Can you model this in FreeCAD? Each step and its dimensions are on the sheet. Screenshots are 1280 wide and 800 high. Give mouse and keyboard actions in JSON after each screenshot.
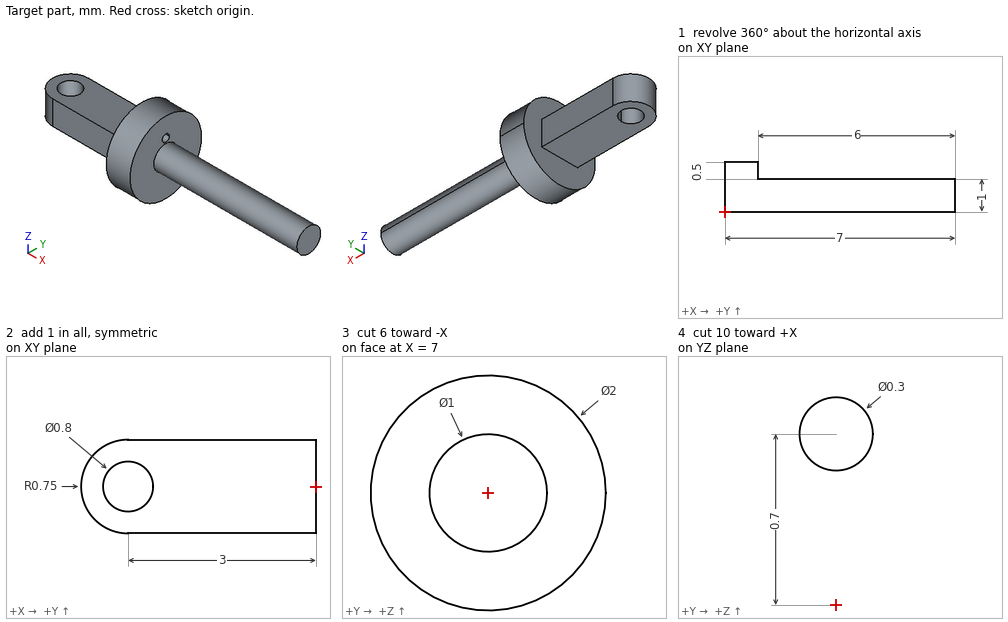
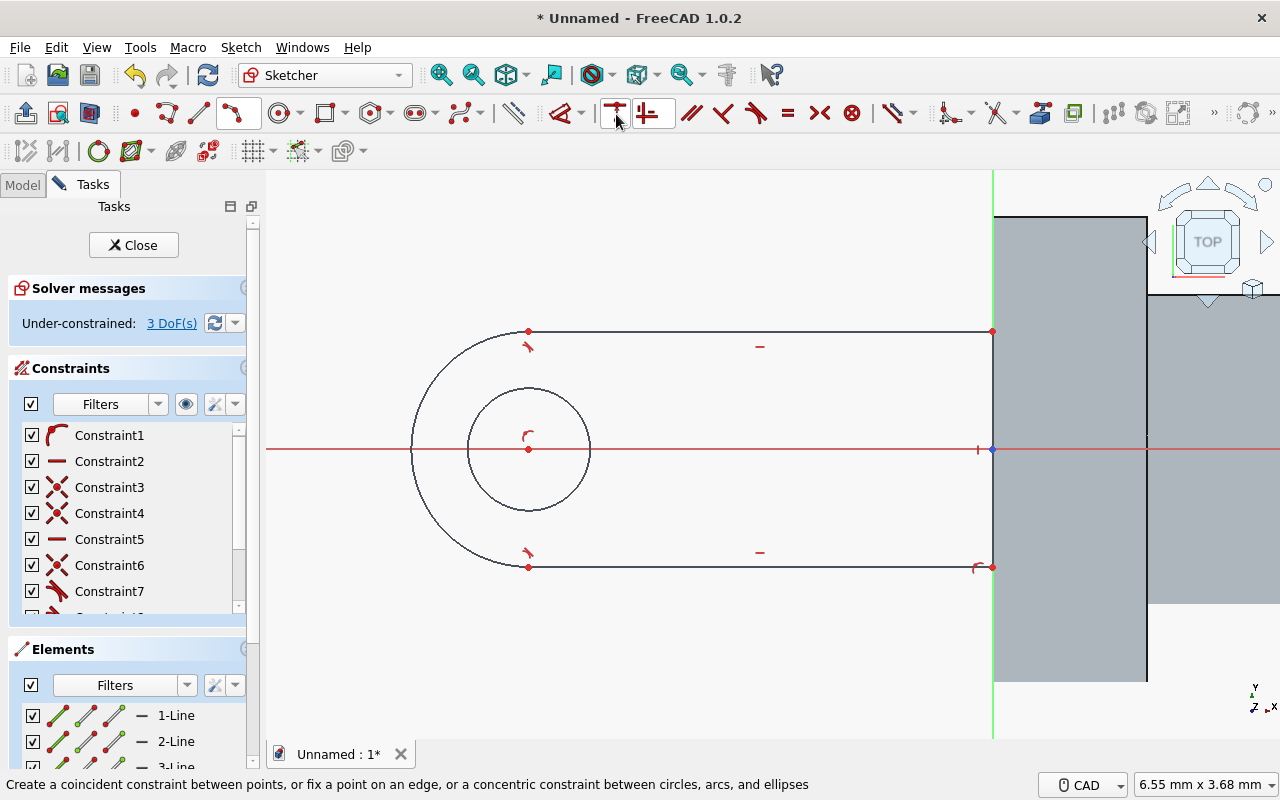
{"action": "left_click", "coordinate": [560, 114]}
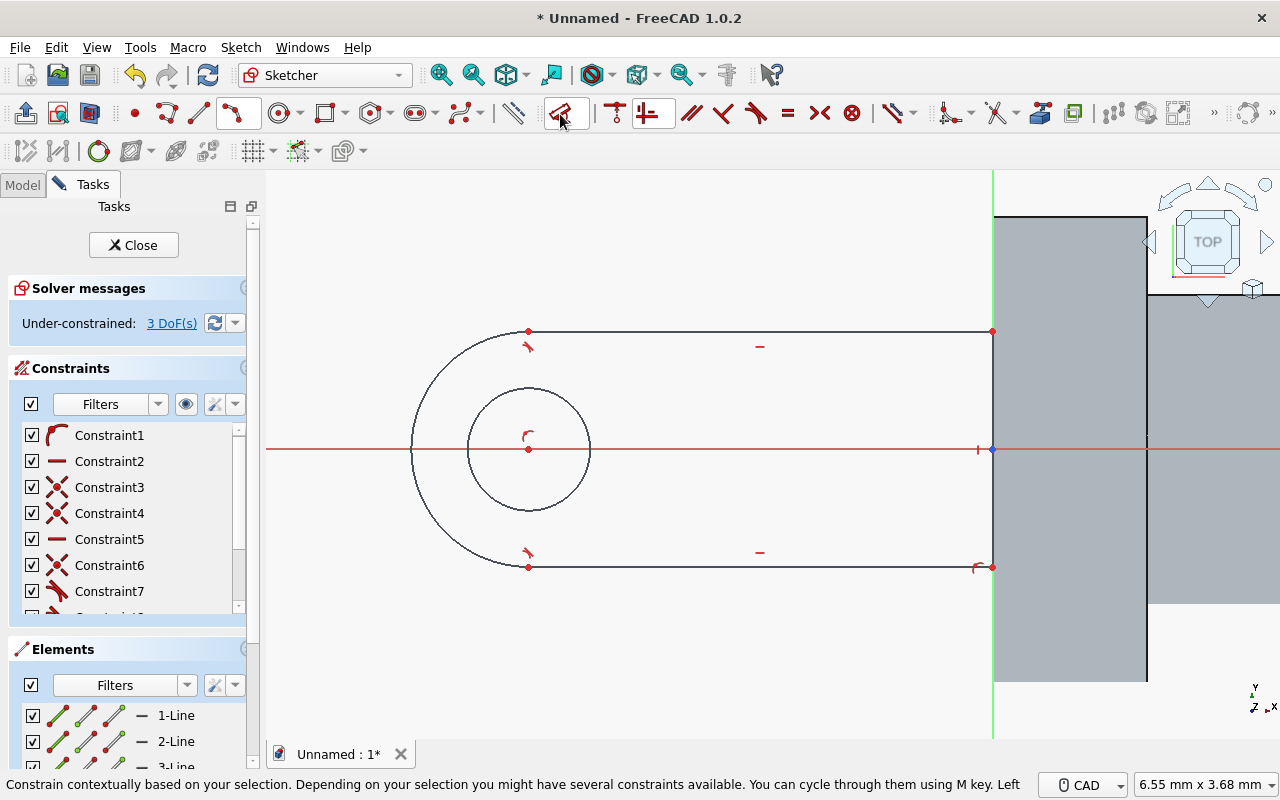
{"action": "left_click", "coordinate": [434, 380]}
{"action": "left_click", "coordinate": [408, 361]}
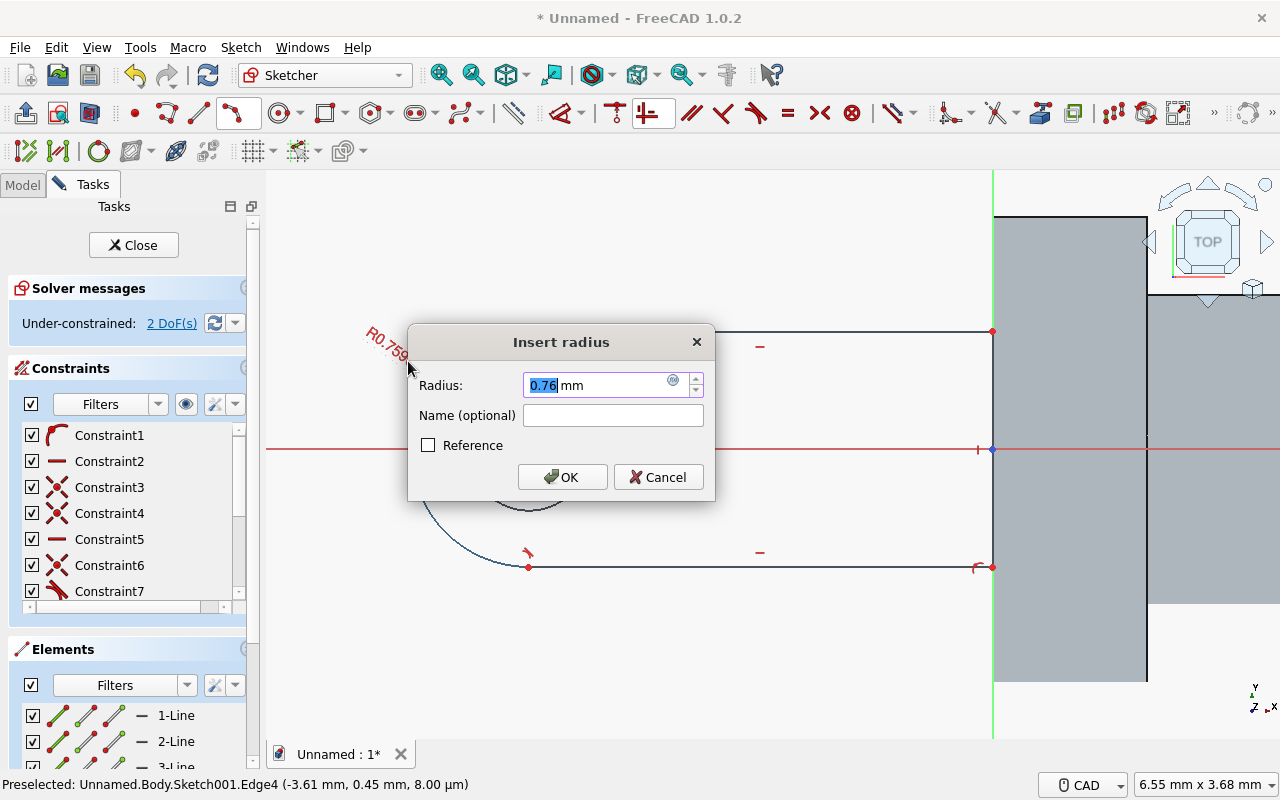
{"action": "type", "text": "0.75"}
{"action": "key", "text": "Return"}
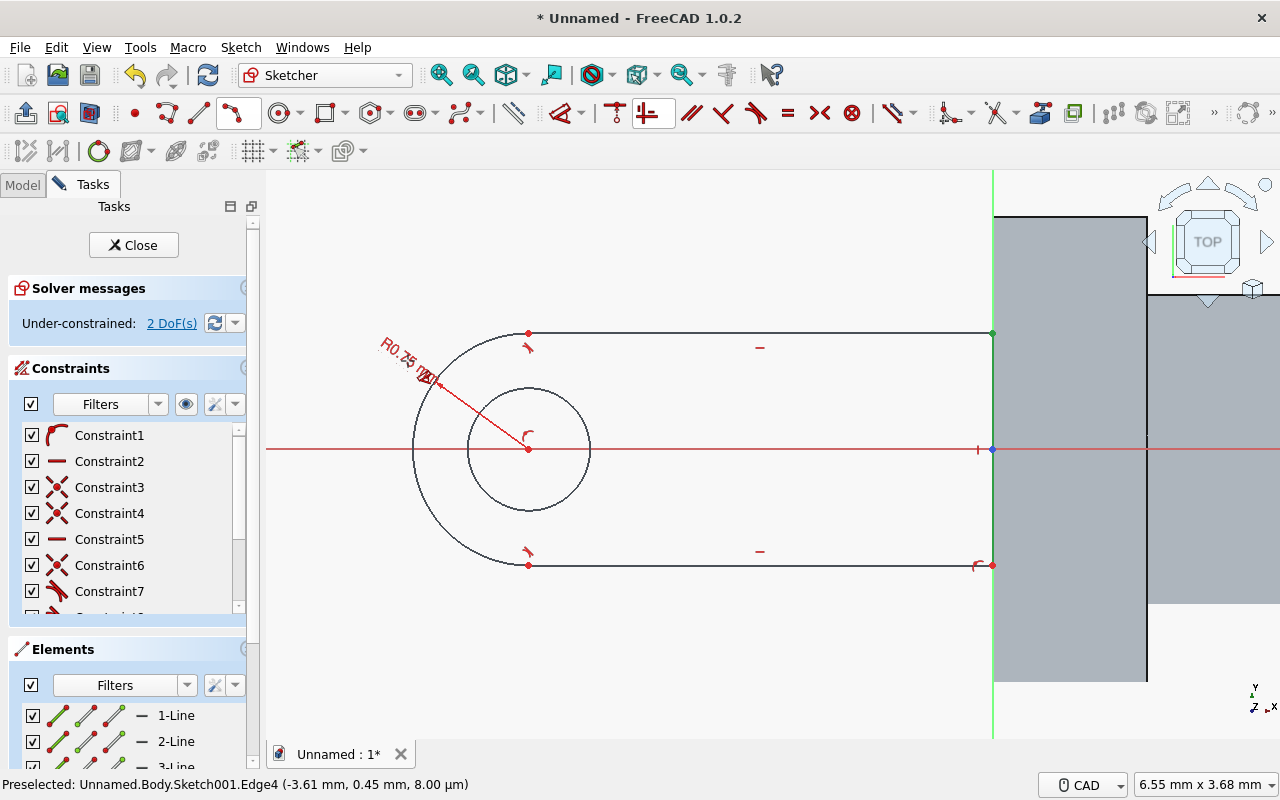
{"action": "left_click", "coordinate": [572, 406]}
{"action": "left_click", "coordinate": [595, 383]}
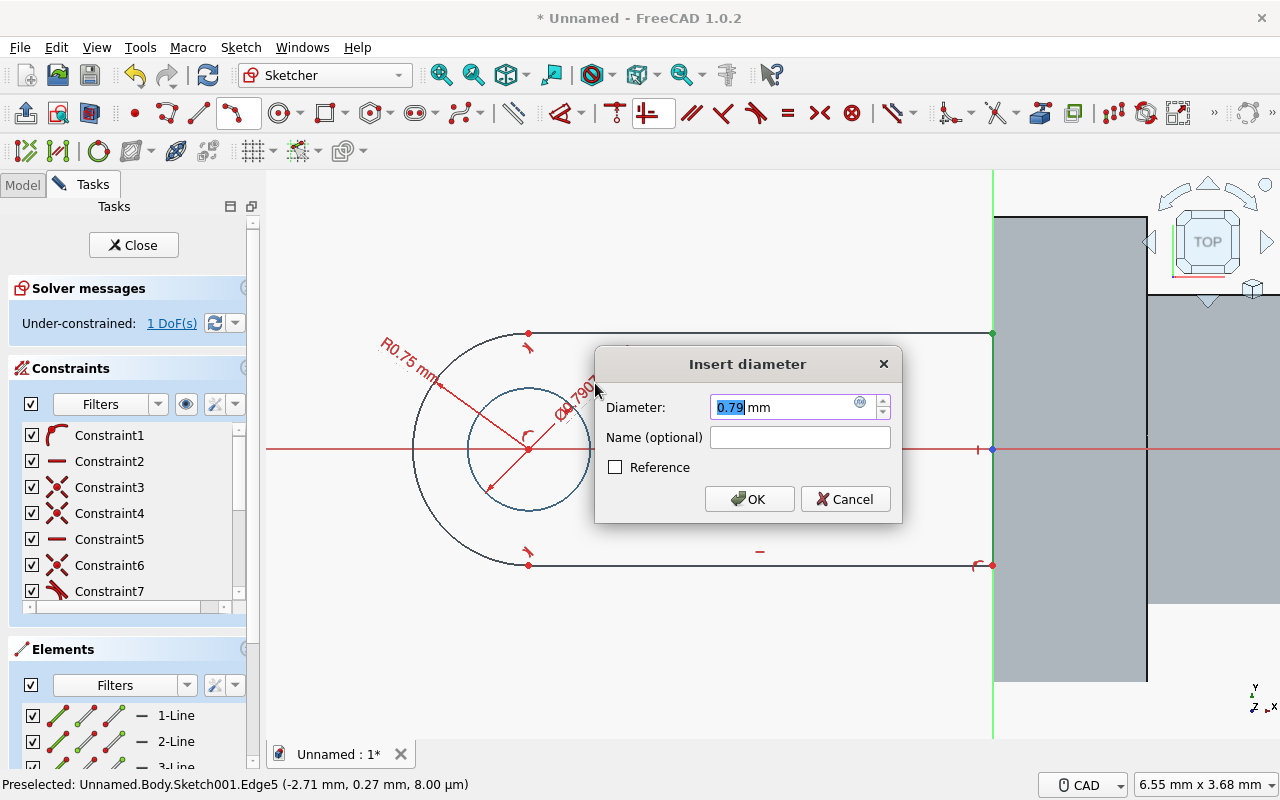
{"action": "type", "text": "0.8"}
{"action": "key", "text": "Return"}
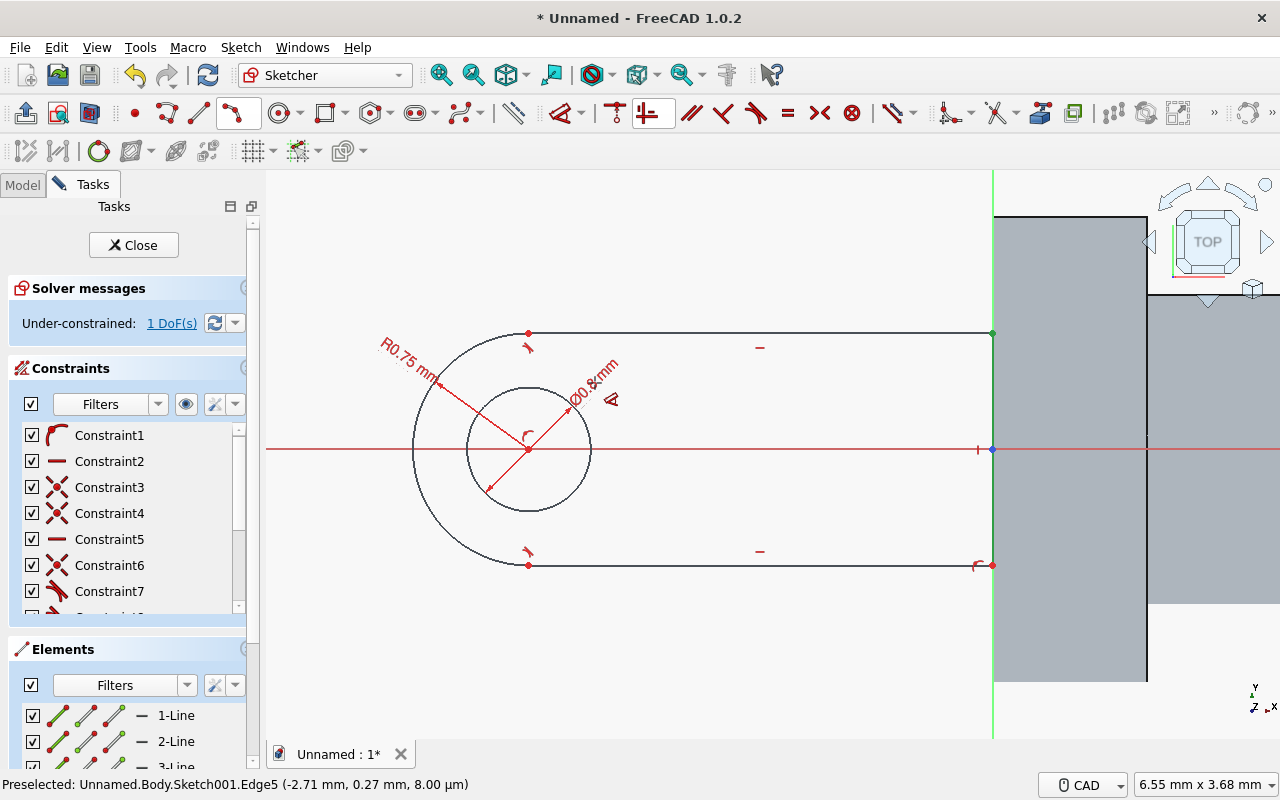
{"action": "left_click", "coordinate": [668, 566]}
{"action": "left_click", "coordinate": [761, 600]}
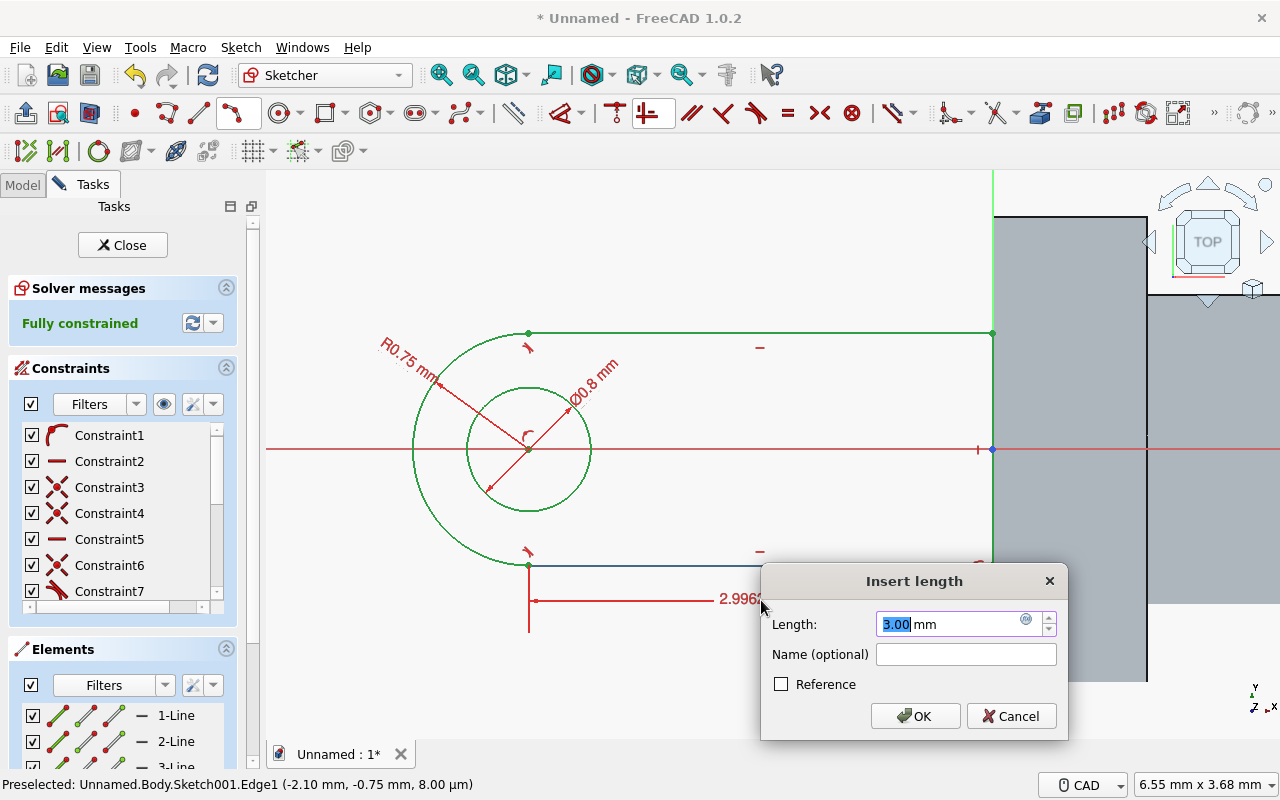
{"action": "type", "text": "3"}
{"action": "key", "text": "Return"}
{"action": "key", "text": "Escape"}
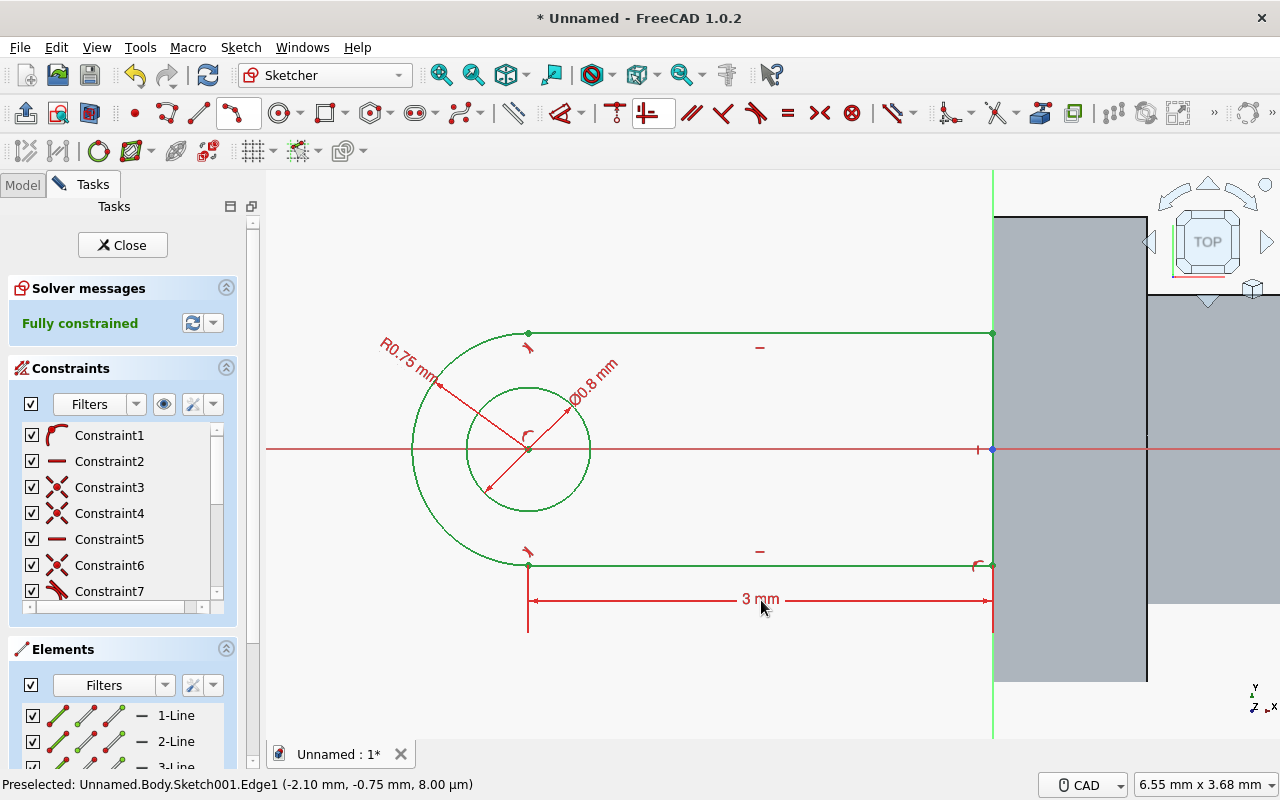
{"action": "left_click", "coordinate": [123, 245]}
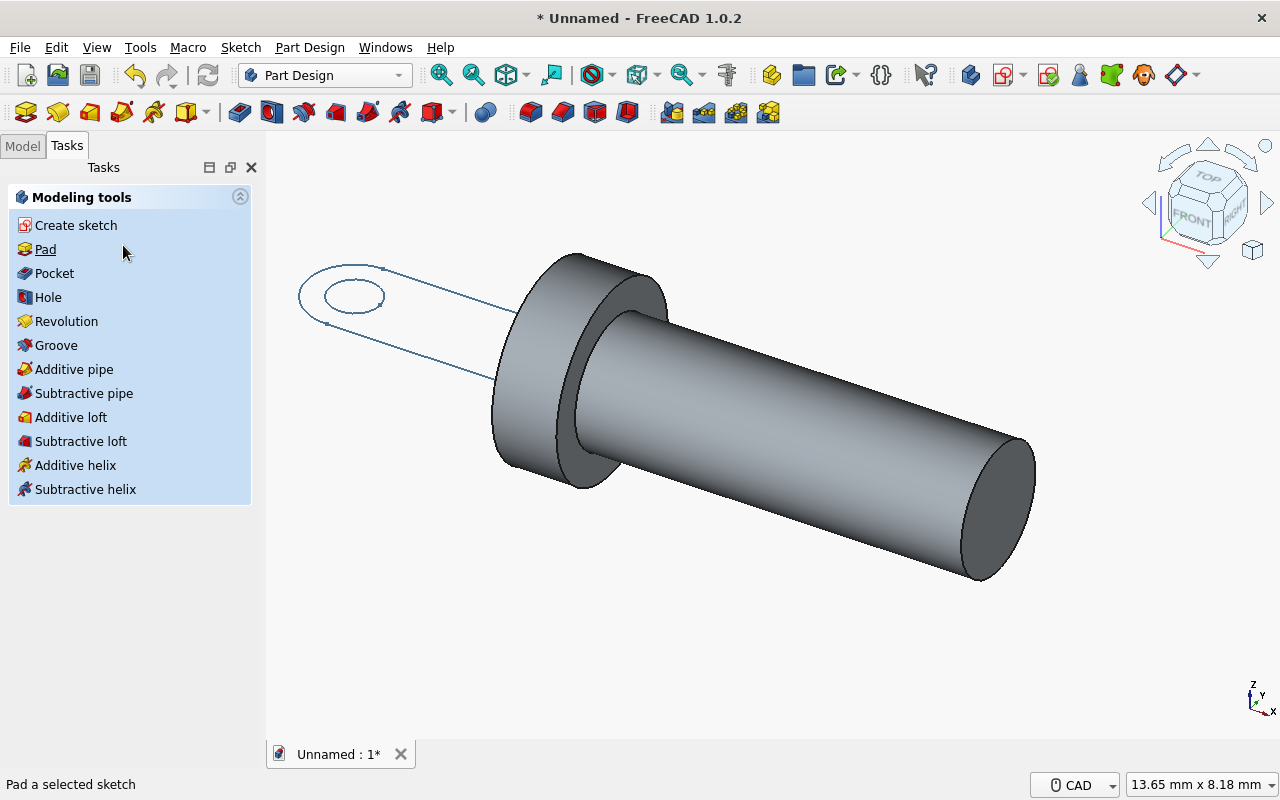
{"action": "left_click", "coordinate": [26, 112]}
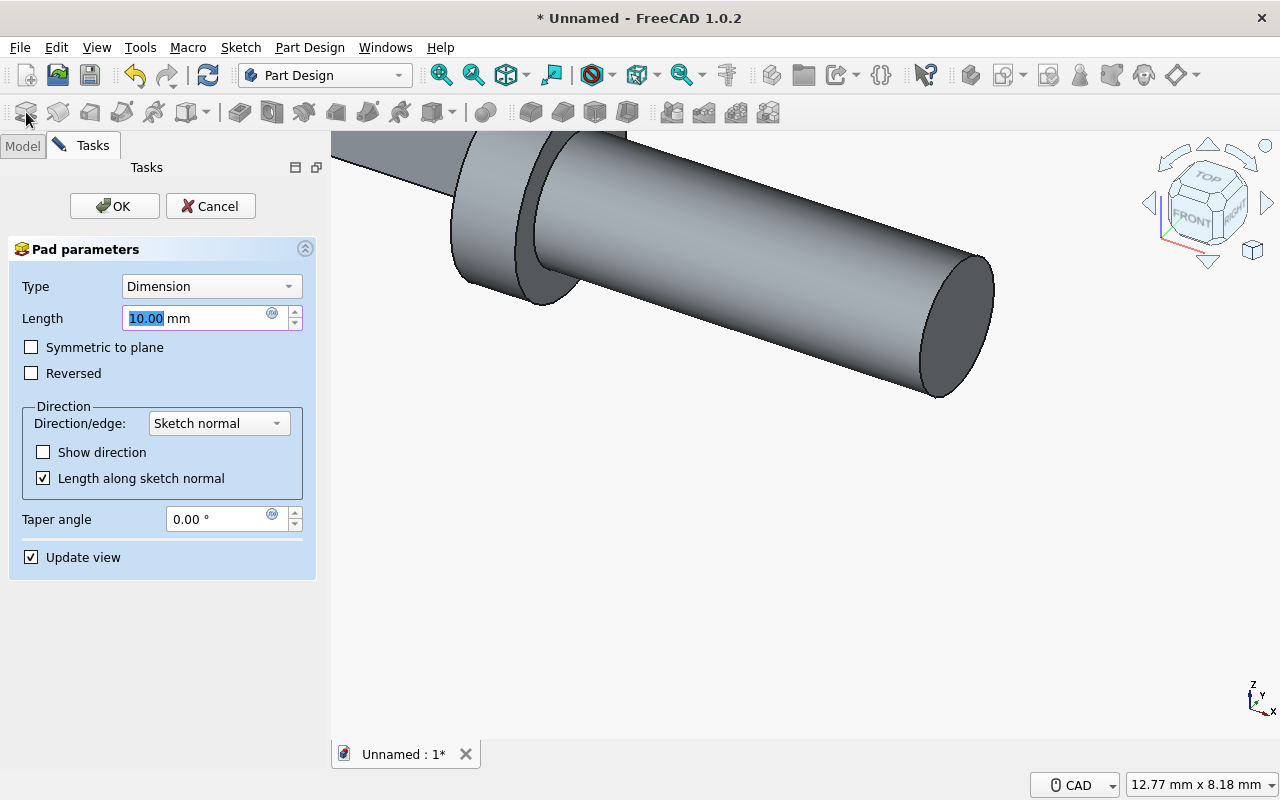
{"action": "type", "text": "1"}
{"action": "key", "text": "Tab"}